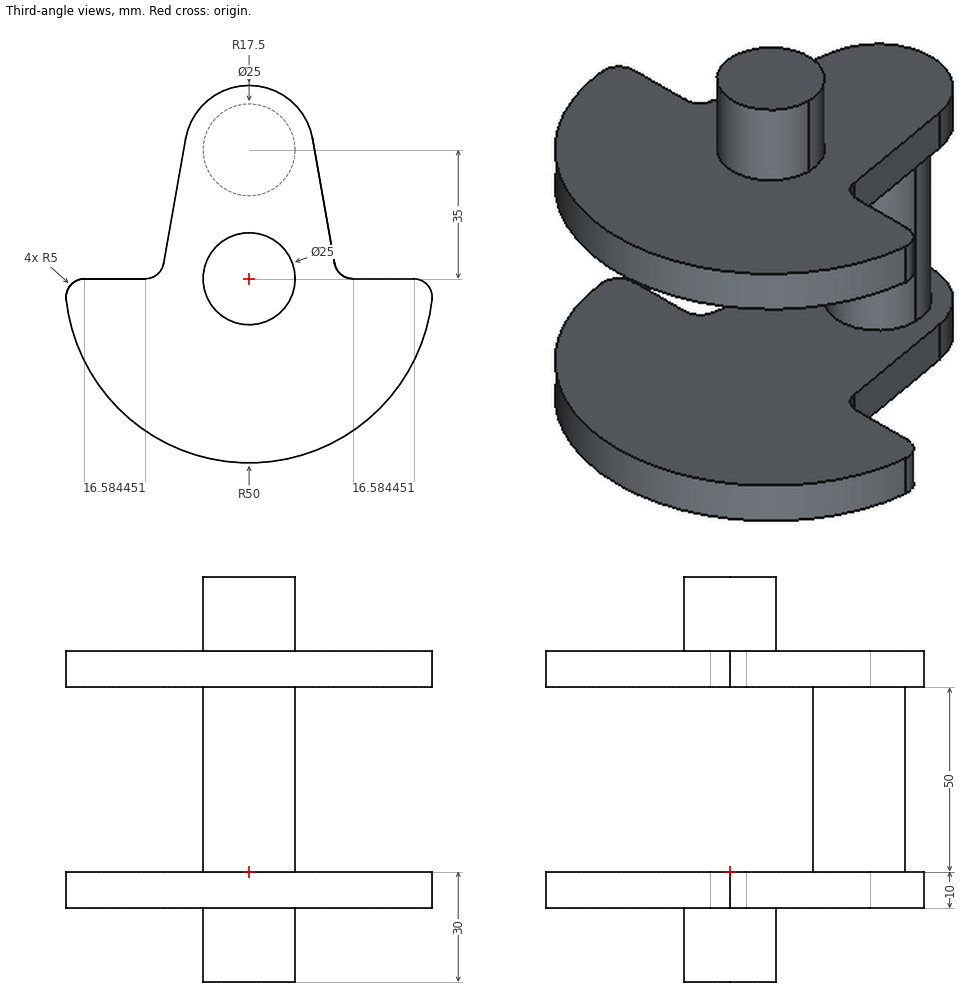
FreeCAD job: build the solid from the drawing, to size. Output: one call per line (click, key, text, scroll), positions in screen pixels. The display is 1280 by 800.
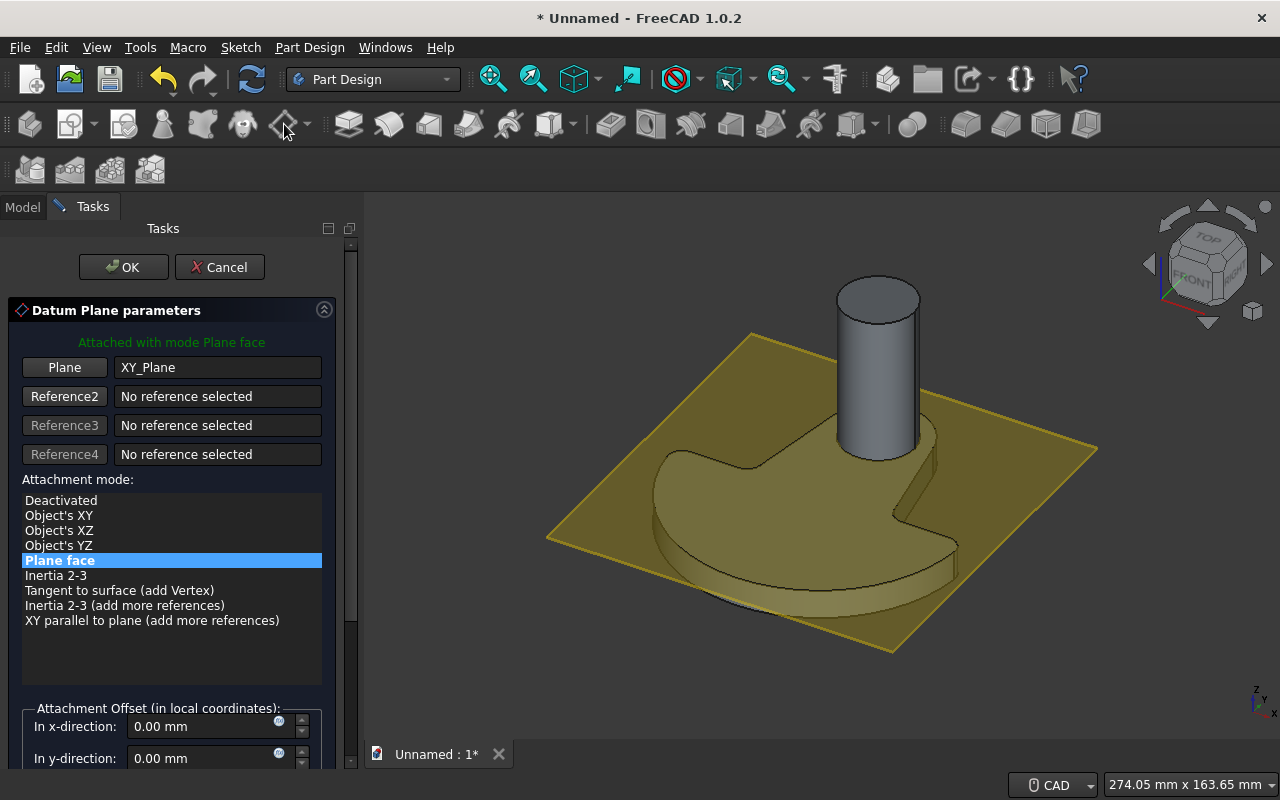
scroll(351, 503, down, 2)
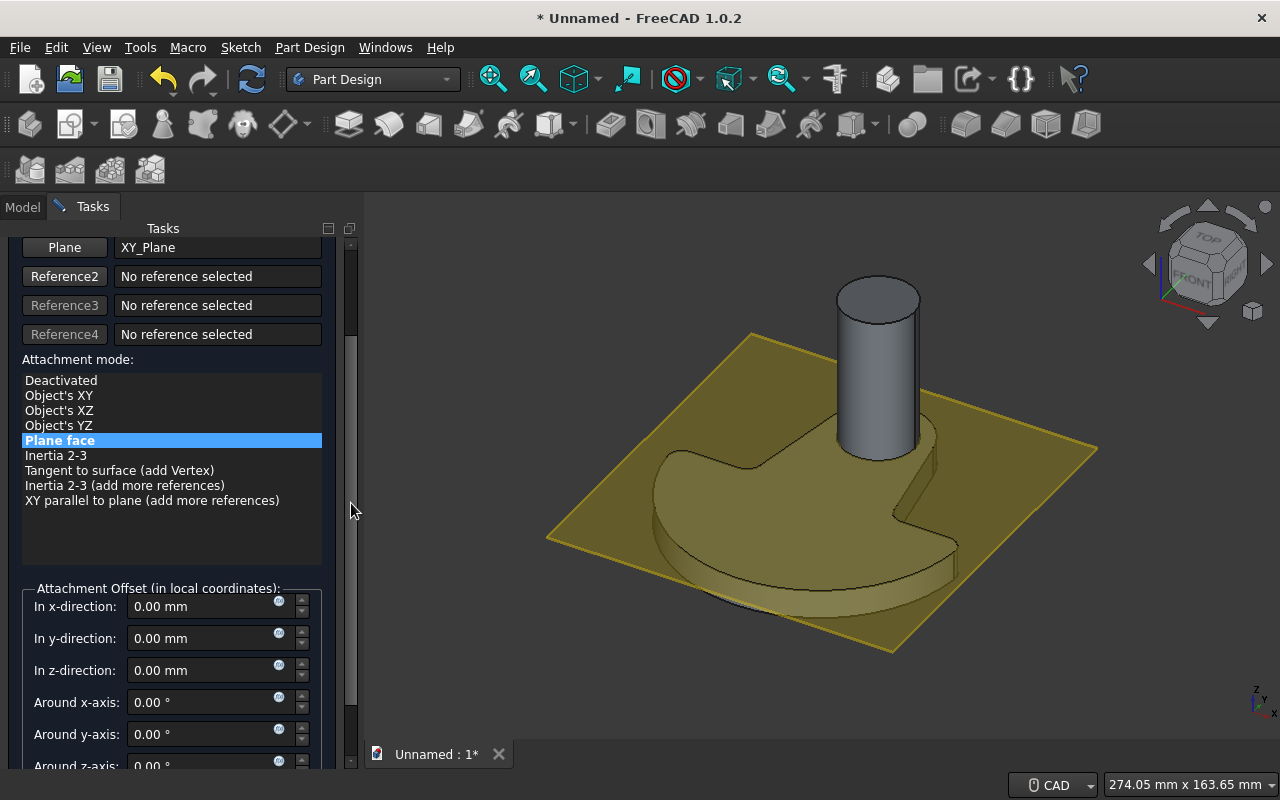
triple_click(210, 670)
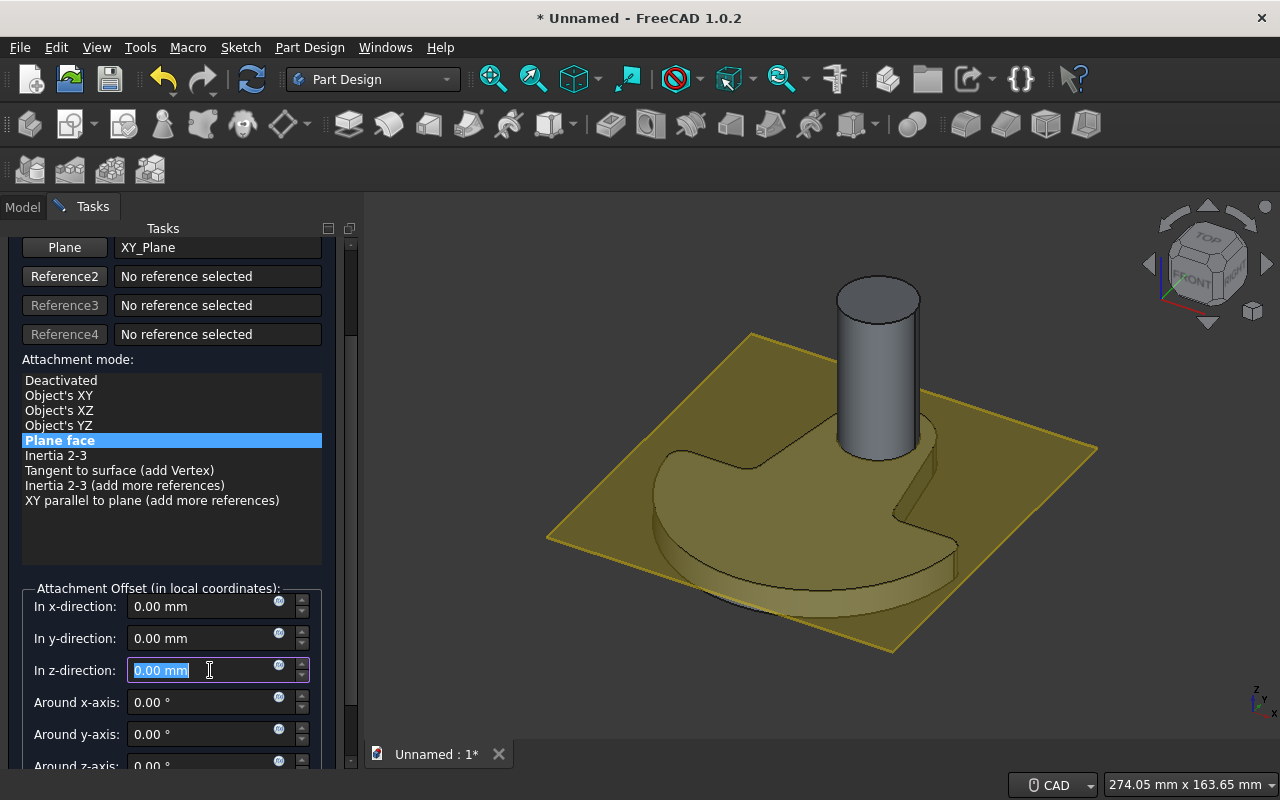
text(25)
key(Tab)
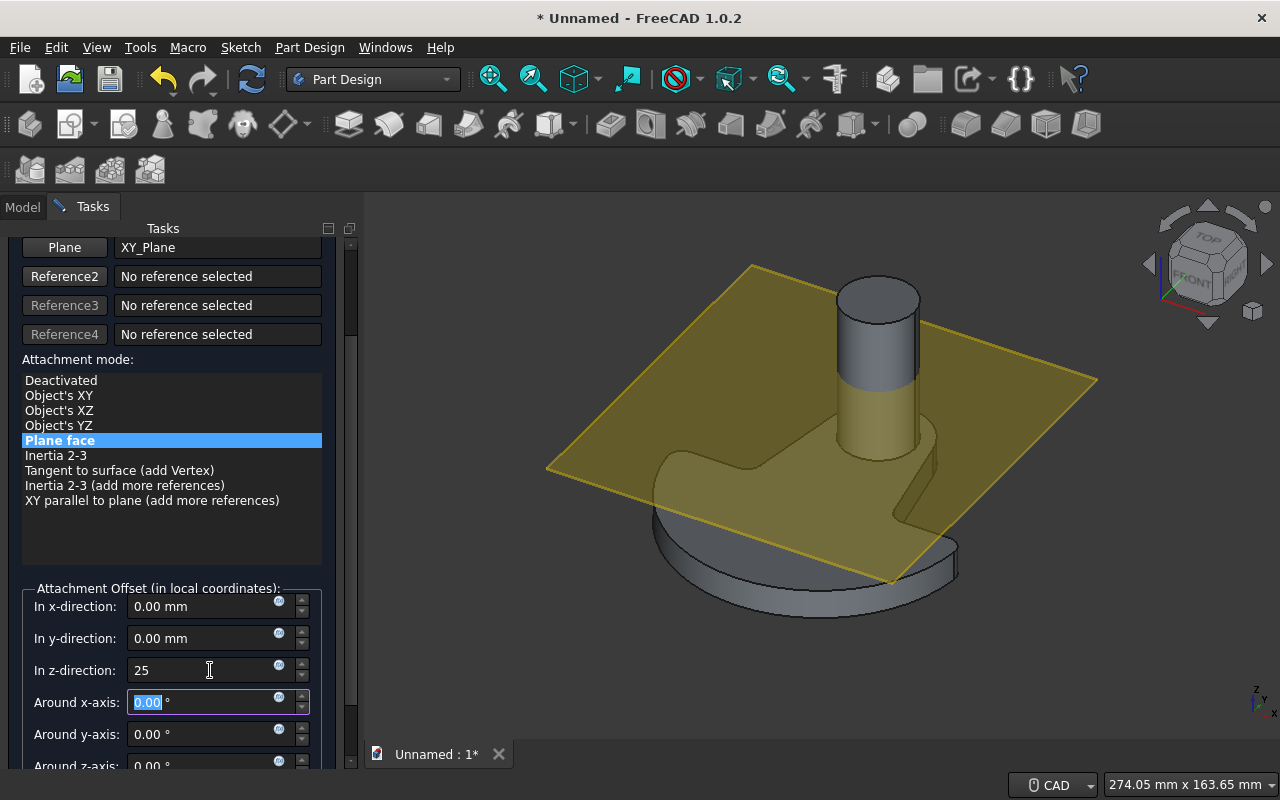
scroll(351, 503, up, 3)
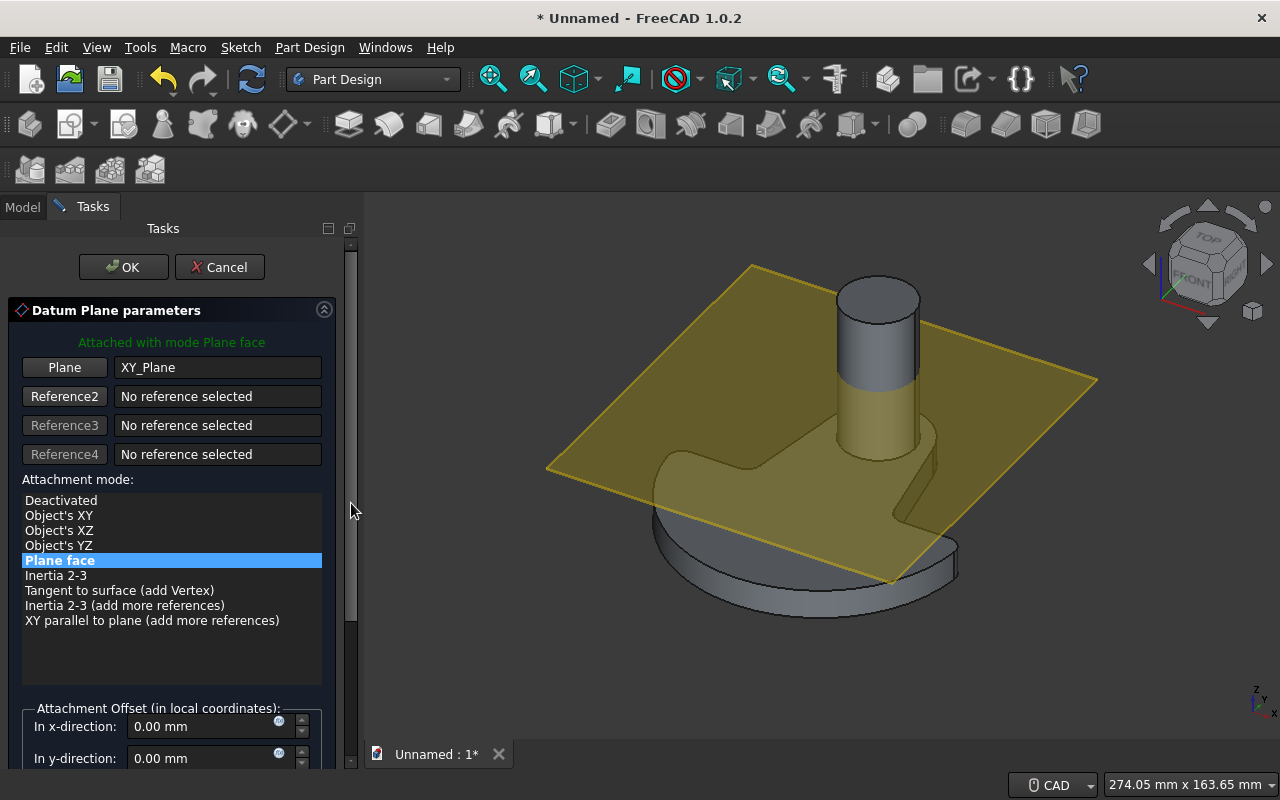
click(124, 267)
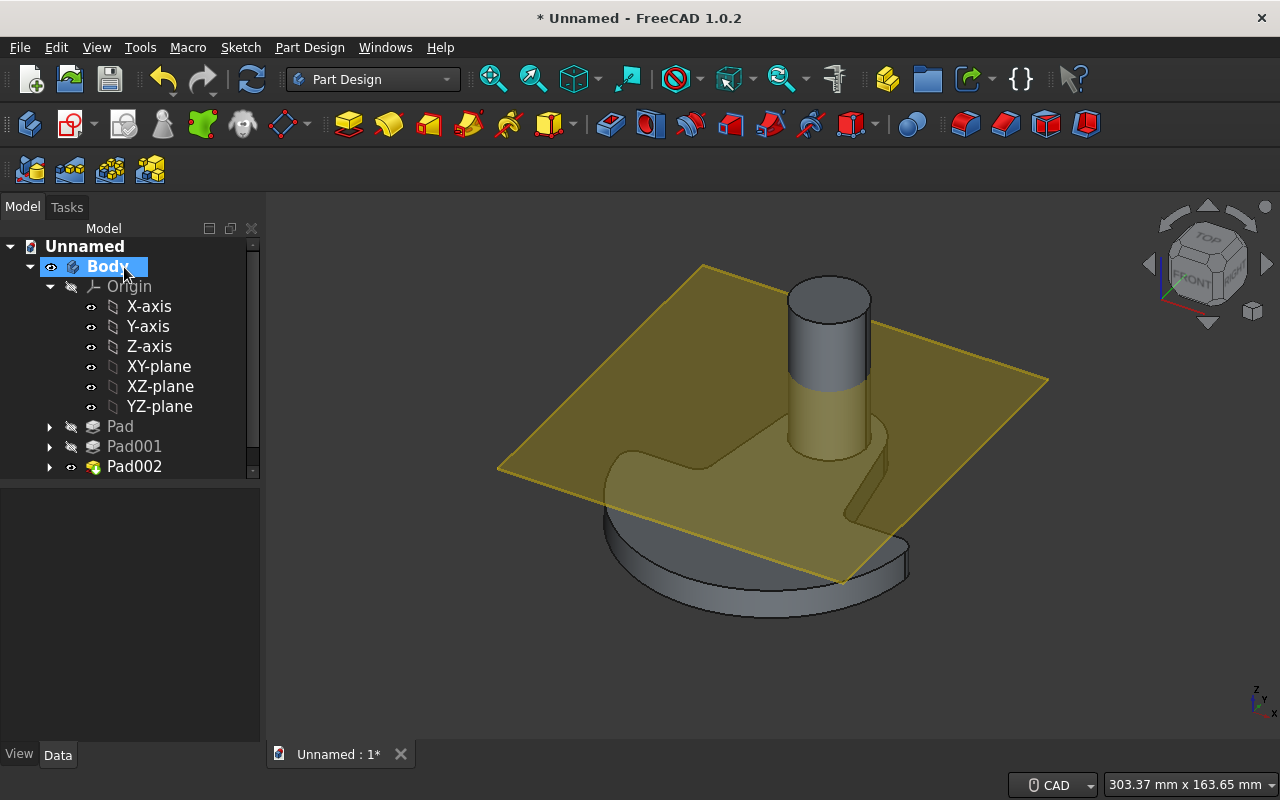
click(116, 427)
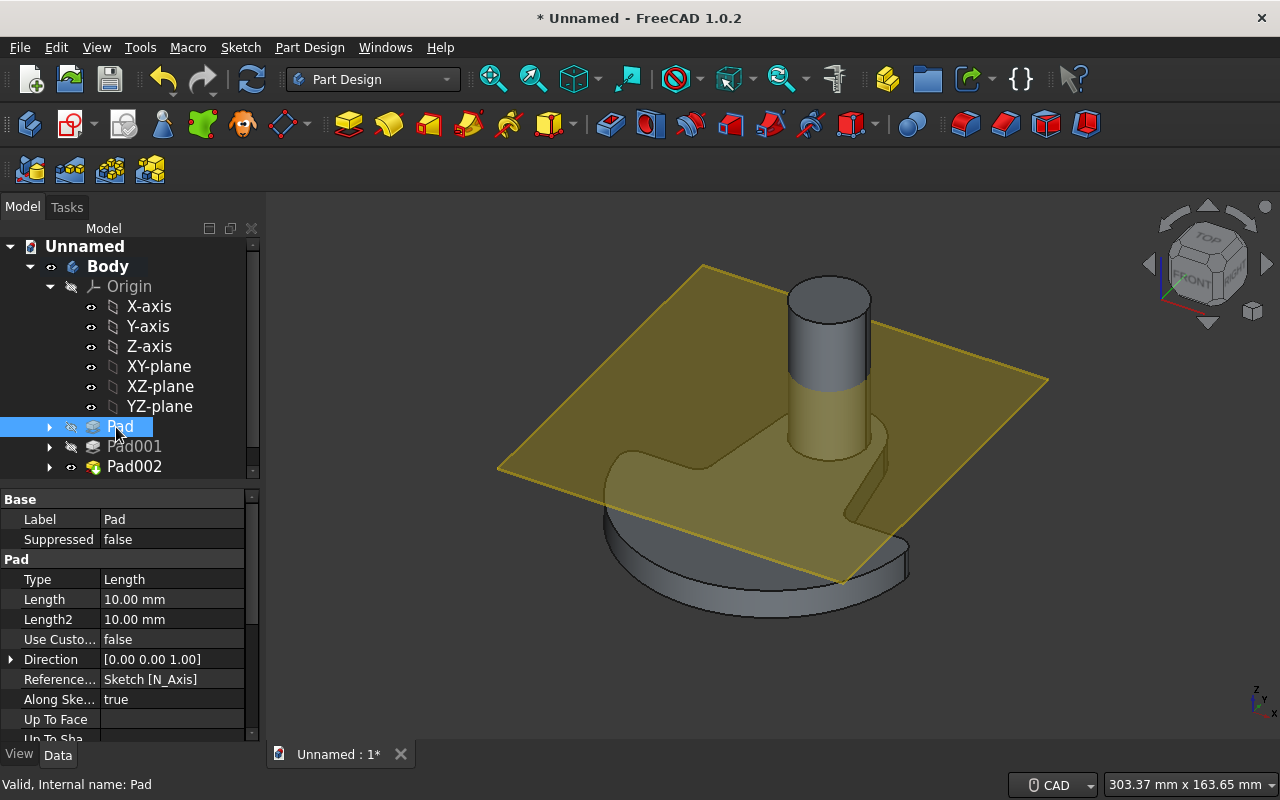
click(116, 447, ctrl)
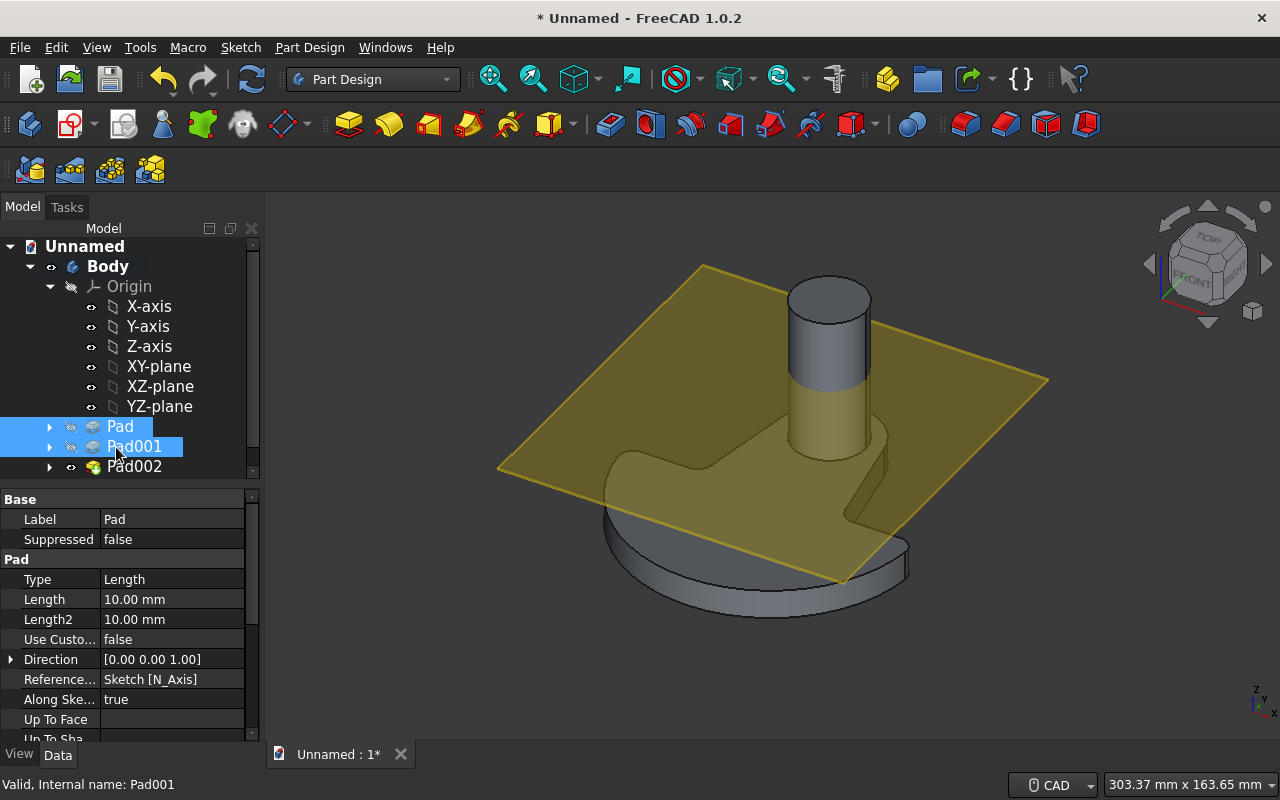
click(30, 170)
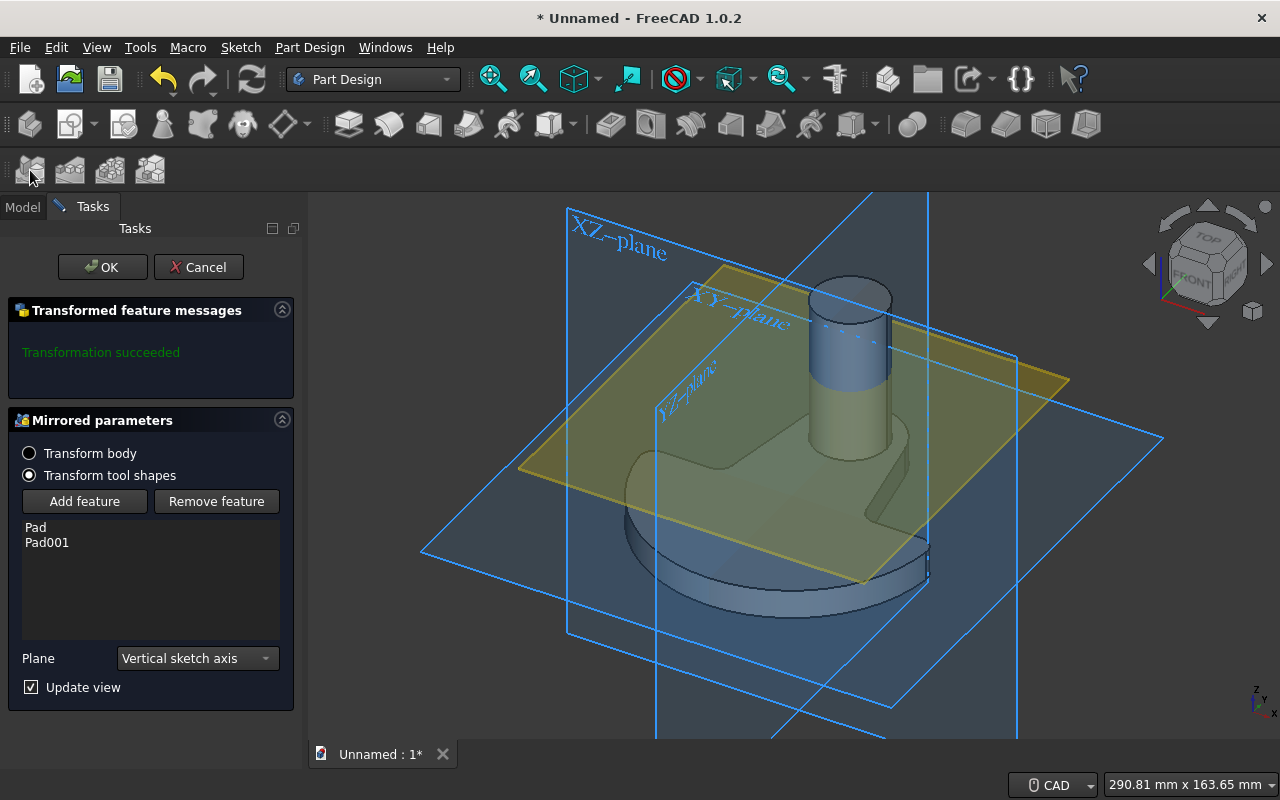
click(198, 658)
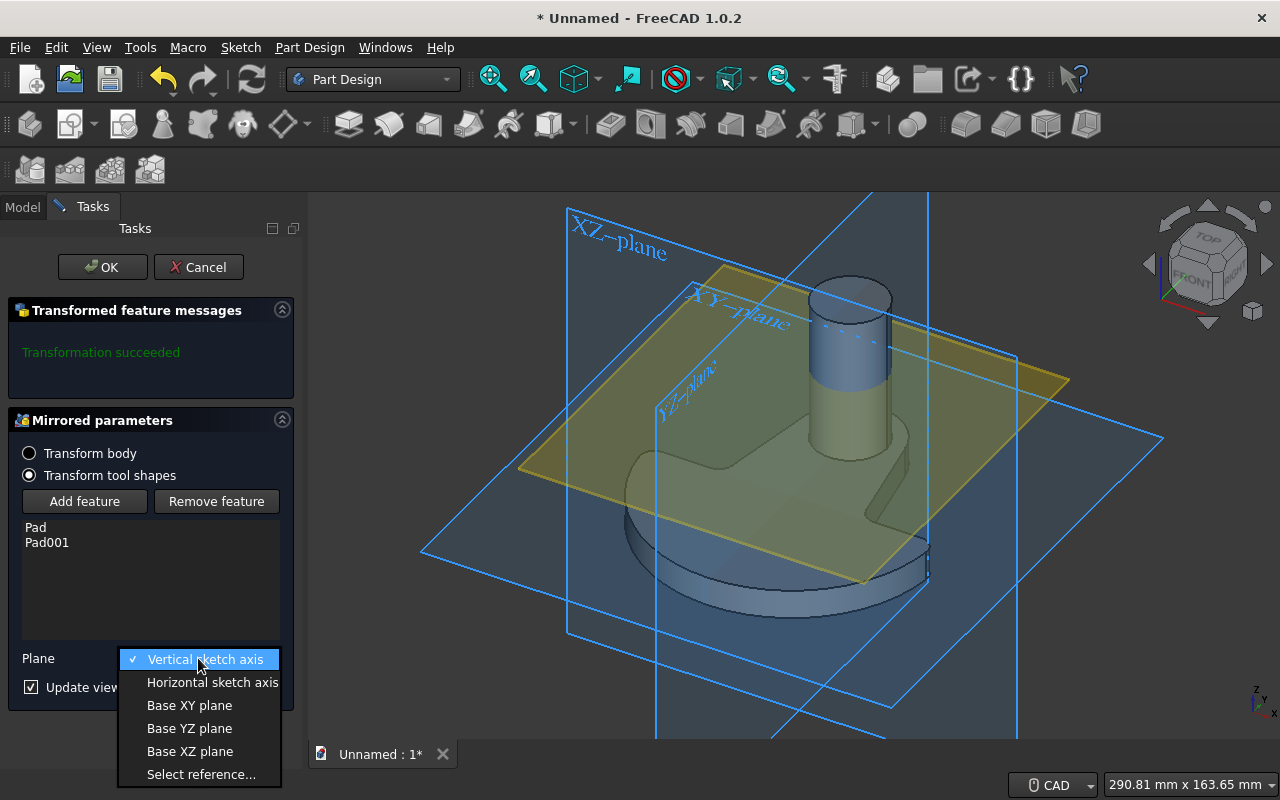
click(198, 774)